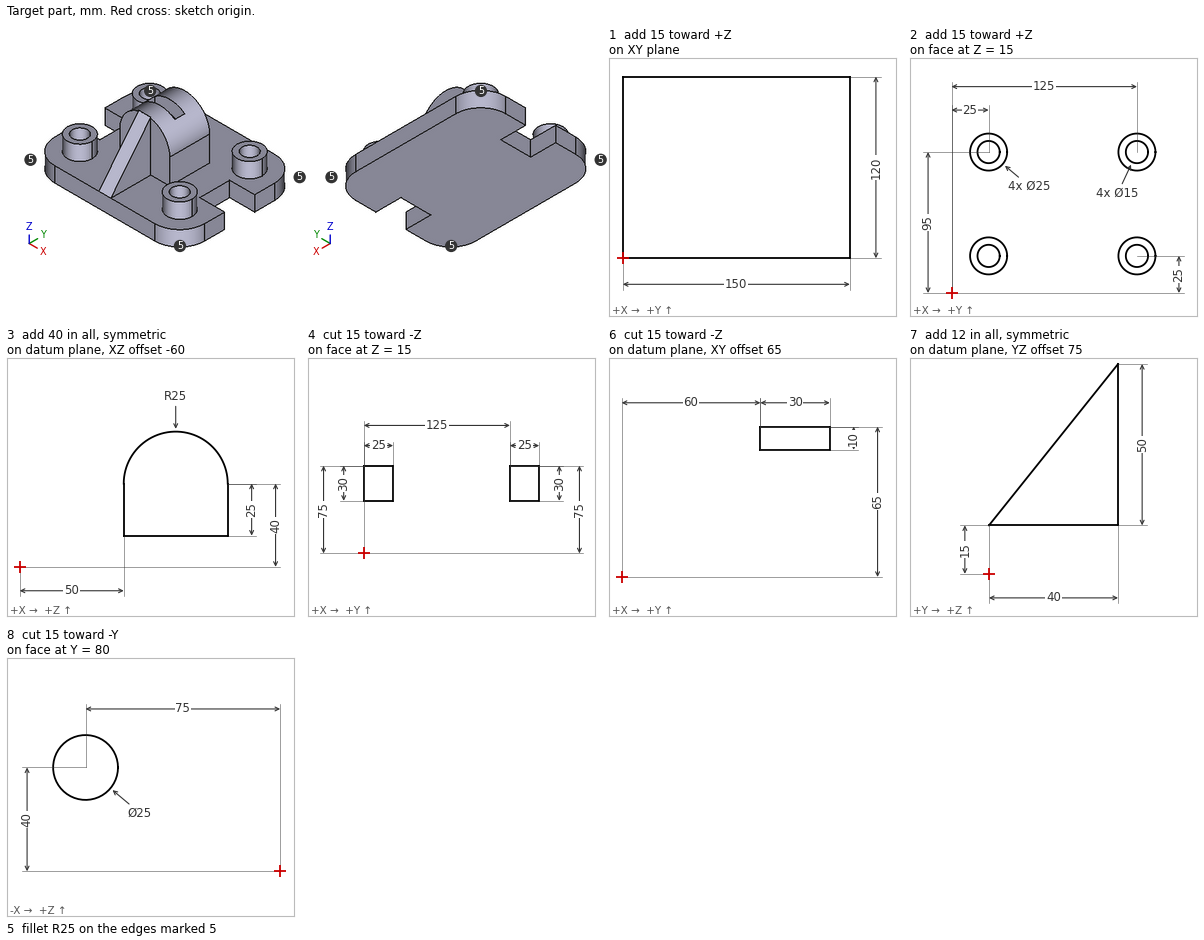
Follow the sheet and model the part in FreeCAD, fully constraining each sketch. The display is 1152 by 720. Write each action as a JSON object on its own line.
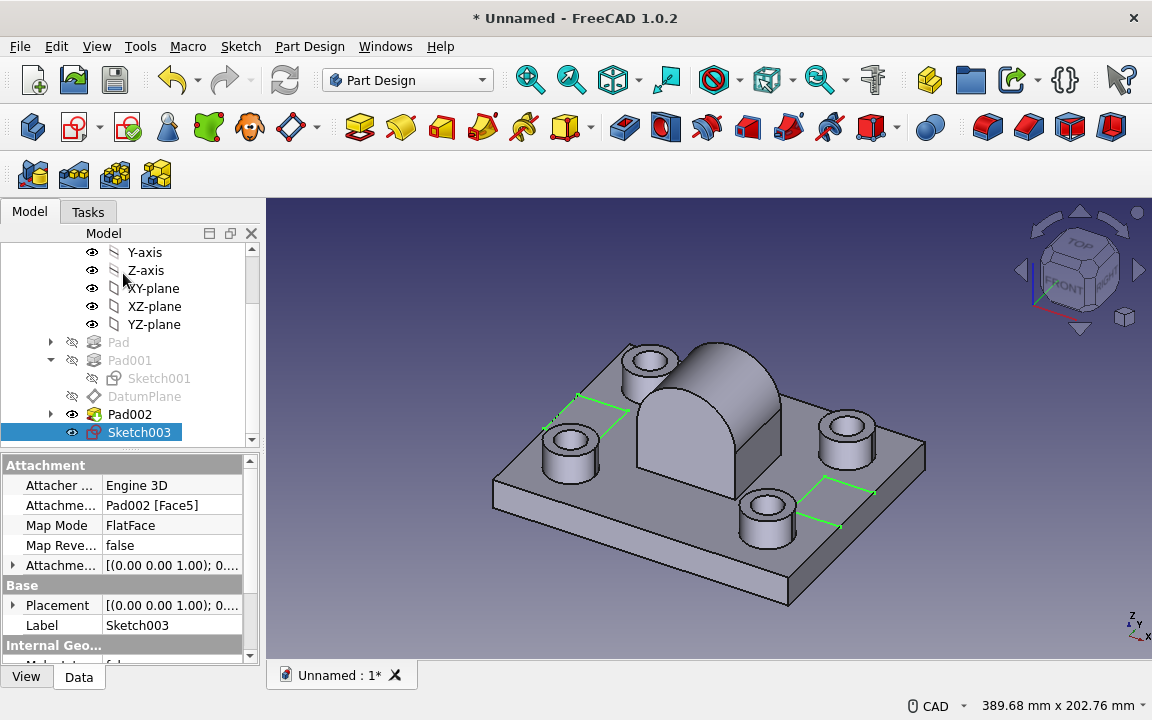
{"action": "left_click", "coordinate": [625, 128]}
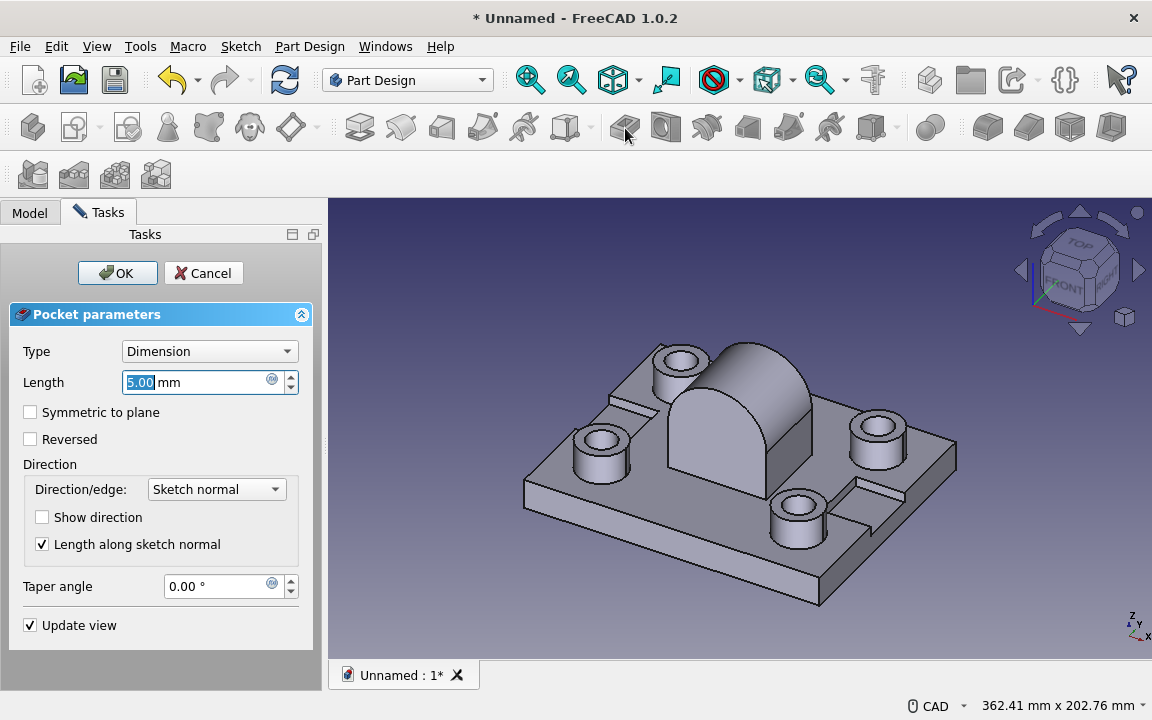
{"action": "type", "text": "15"}
{"action": "key", "text": "Tab"}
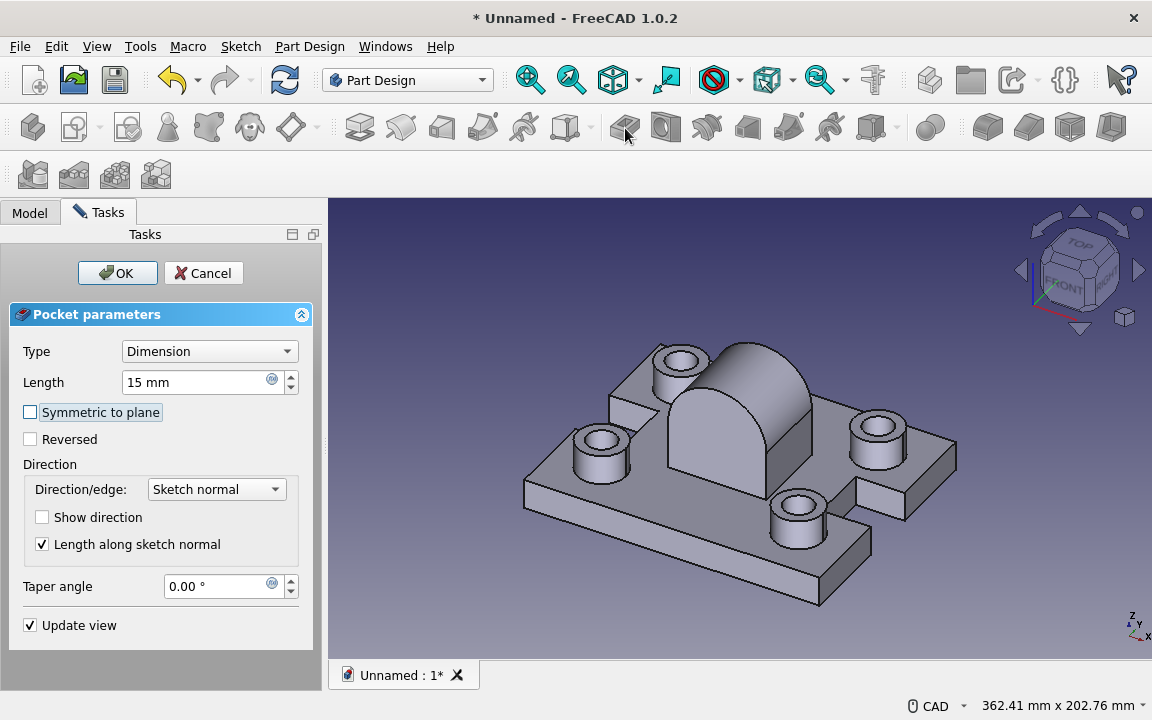
{"action": "left_click", "coordinate": [118, 273]}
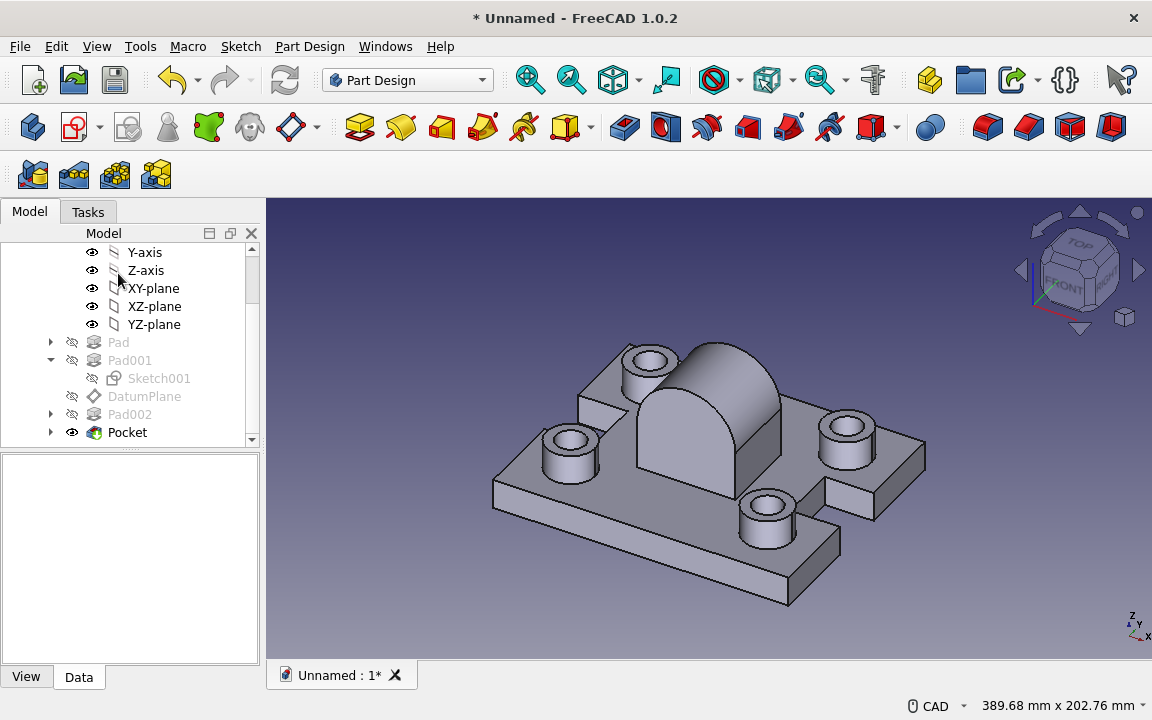
{"action": "left_click", "coordinate": [788, 591]}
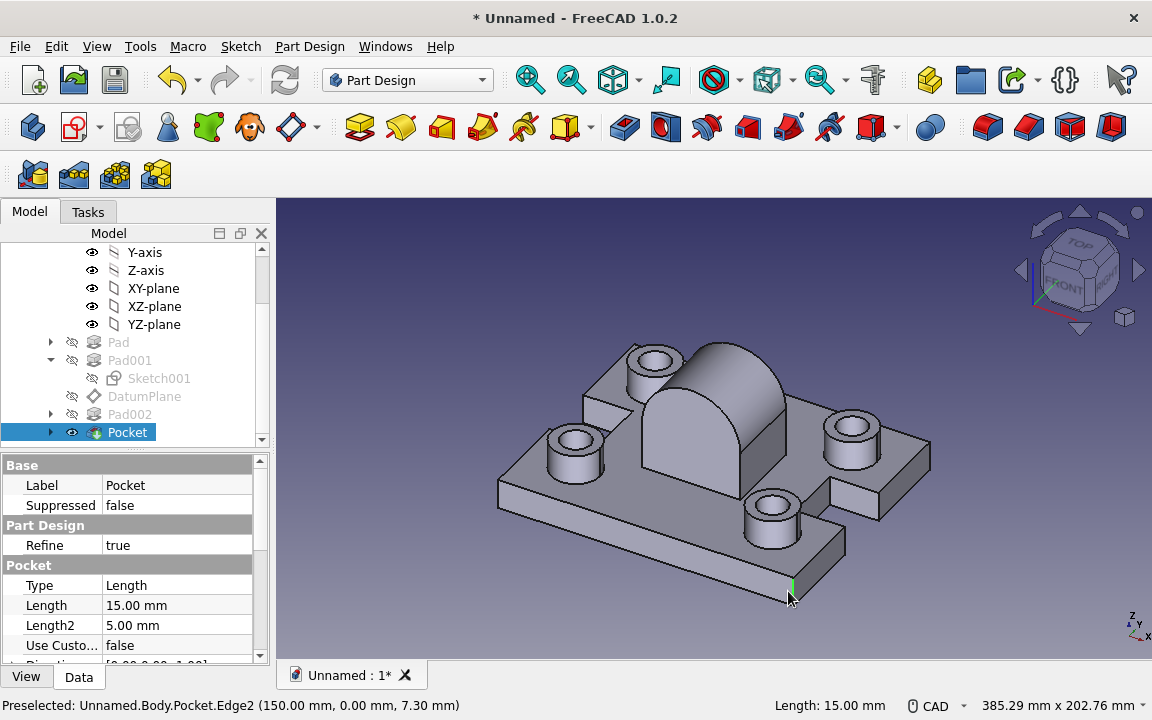
{"action": "key", "text": "0"}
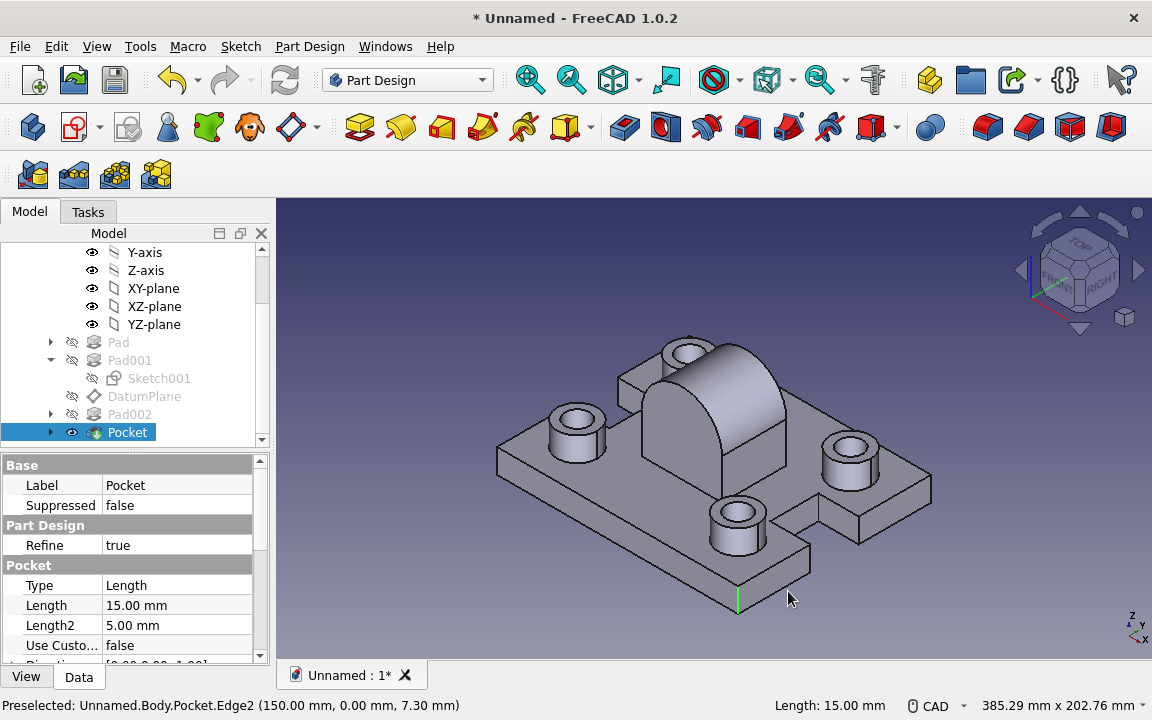
{"action": "key", "text": "2"}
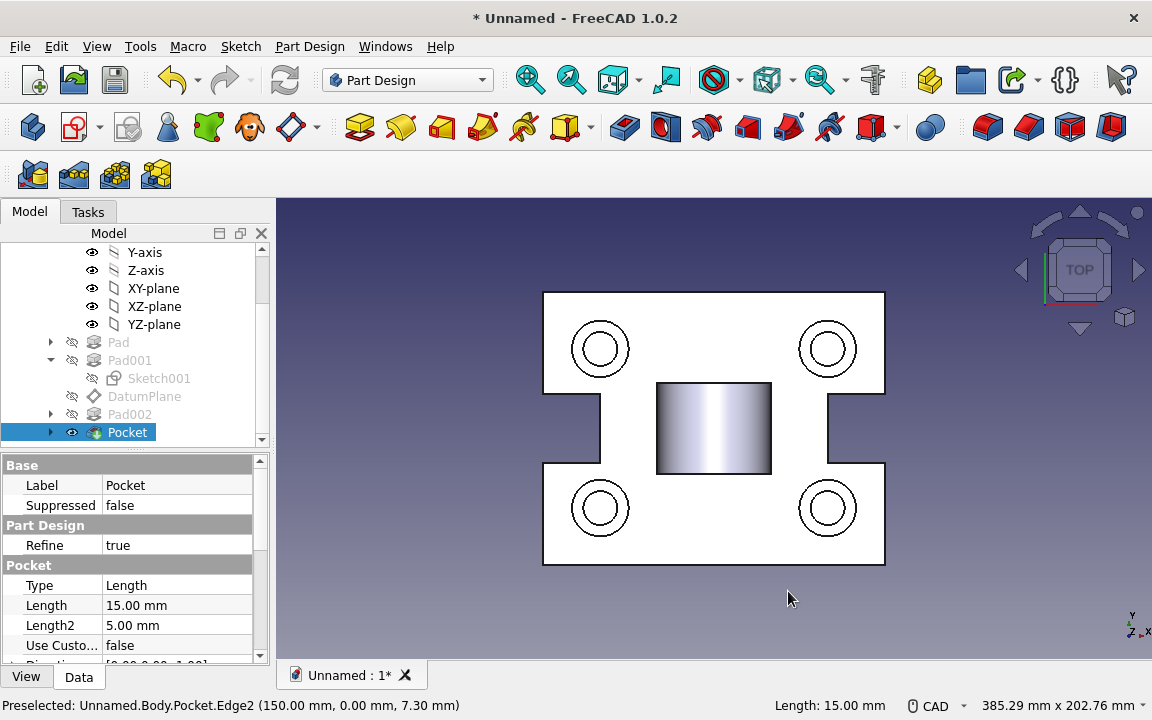
{"action": "key", "text": "1"}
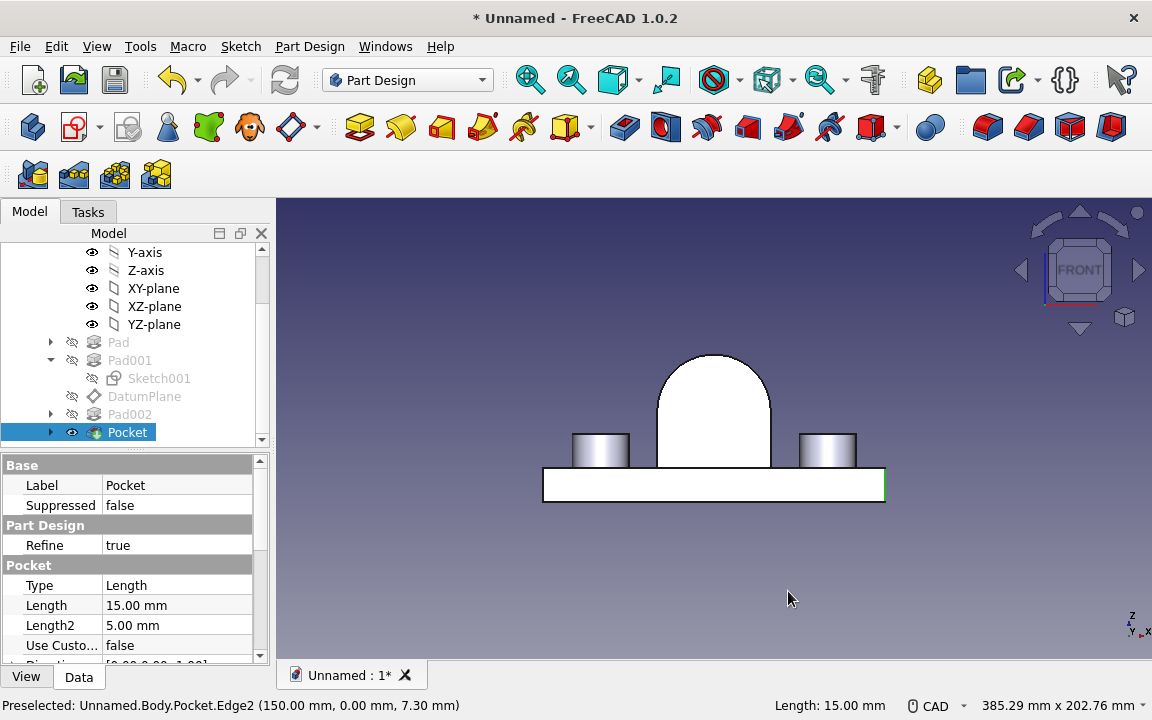
{"action": "key", "text": "v f"}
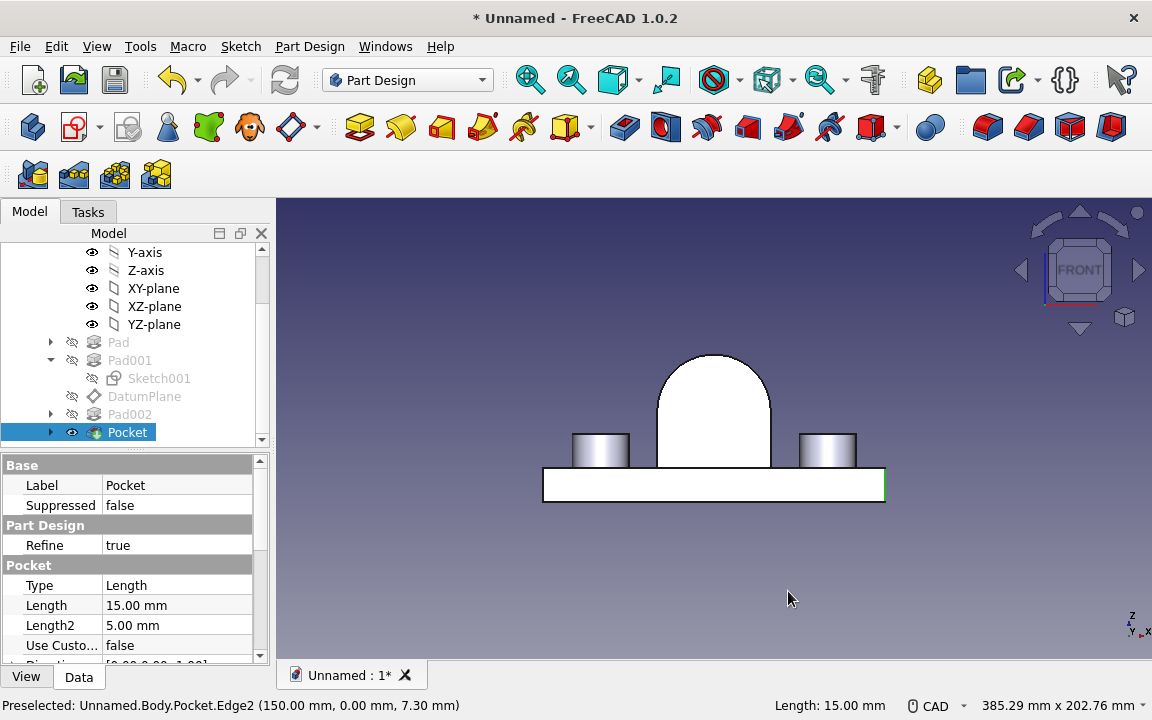
{"action": "left_click", "coordinate": [543, 484], "text": "ctrl"}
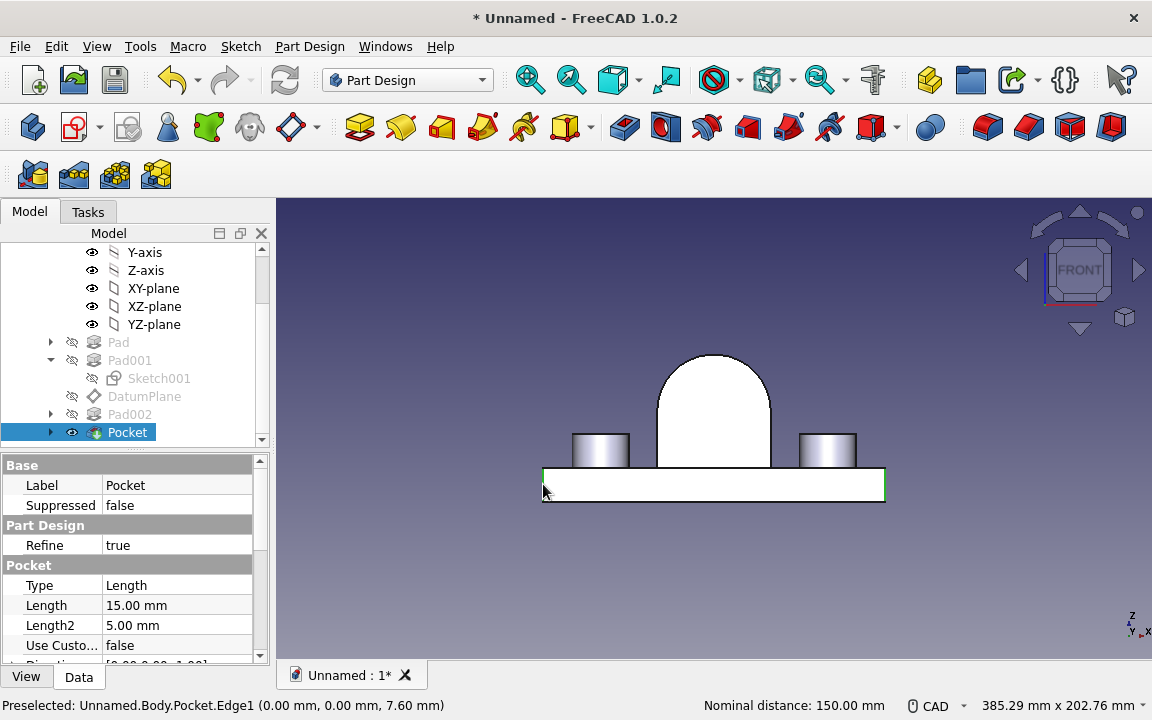
{"action": "key", "text": "3"}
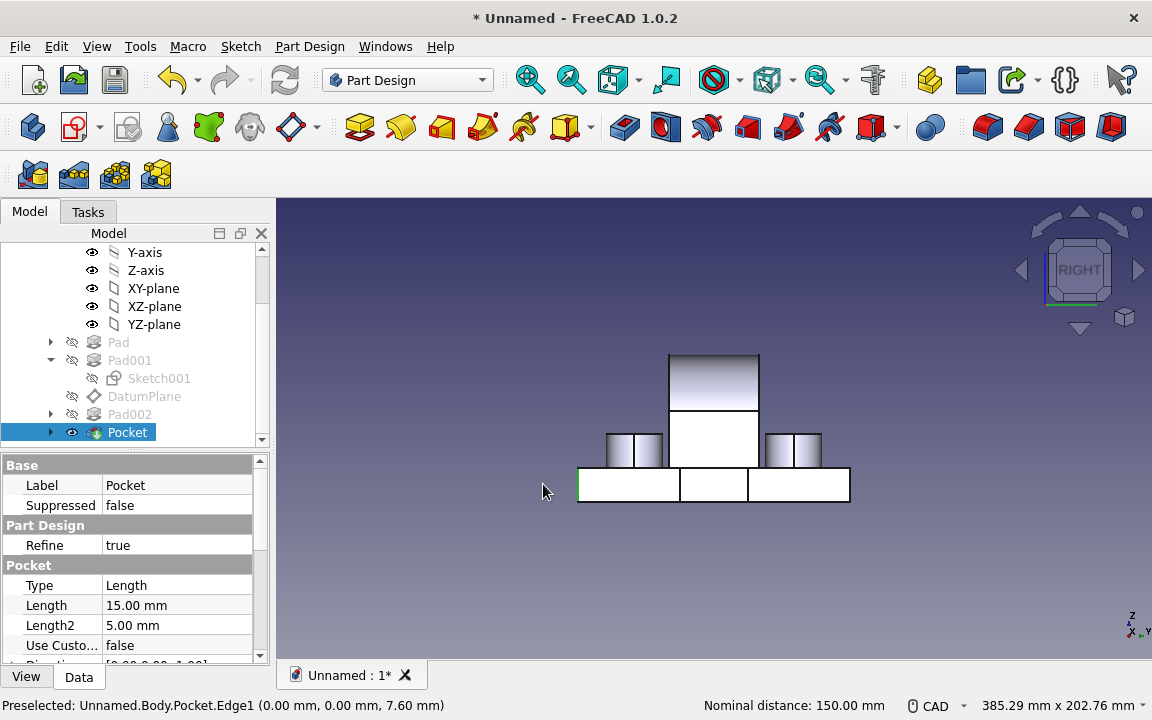
{"action": "key", "text": "v f"}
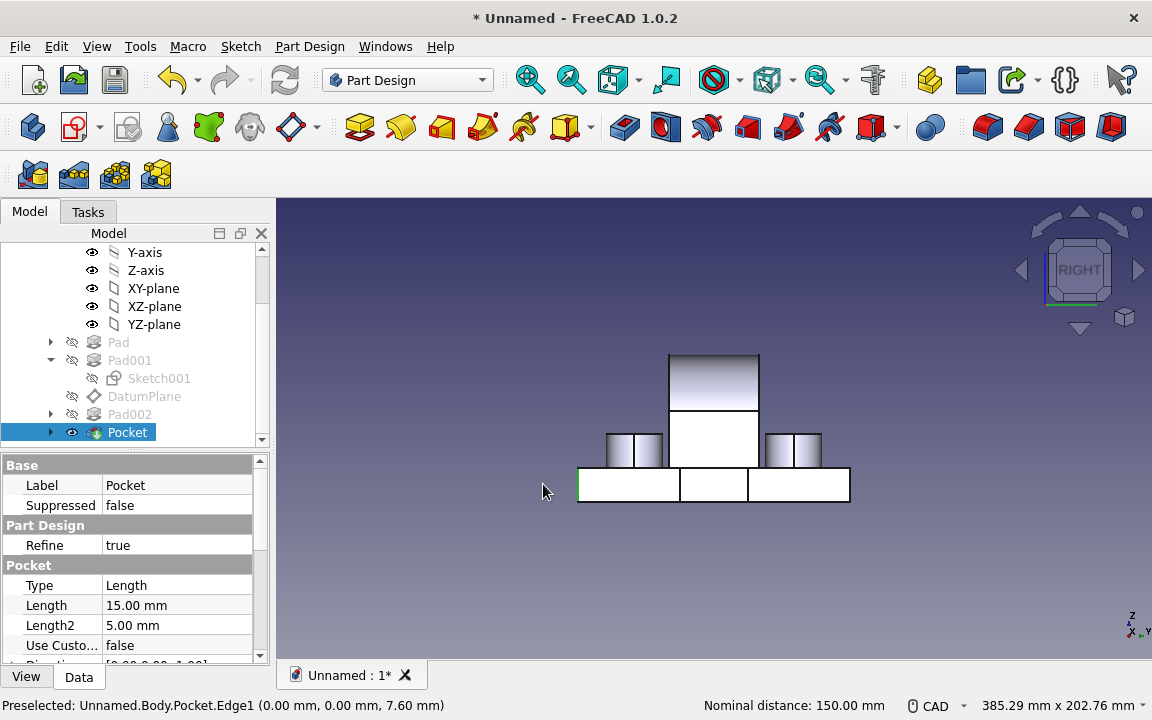
{"action": "left_click", "coordinate": [850, 484], "text": "ctrl"}